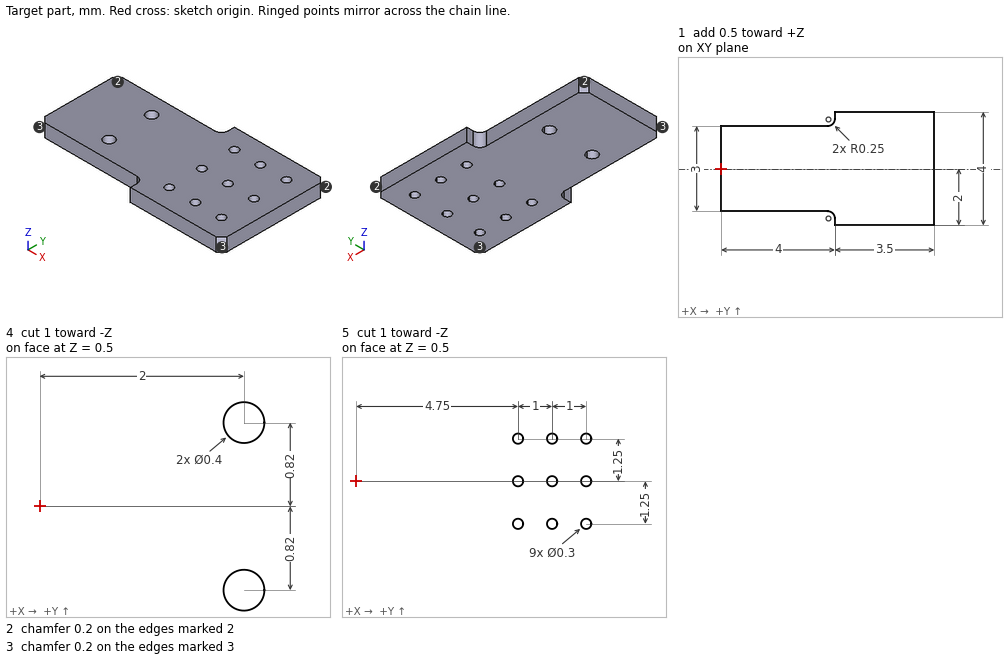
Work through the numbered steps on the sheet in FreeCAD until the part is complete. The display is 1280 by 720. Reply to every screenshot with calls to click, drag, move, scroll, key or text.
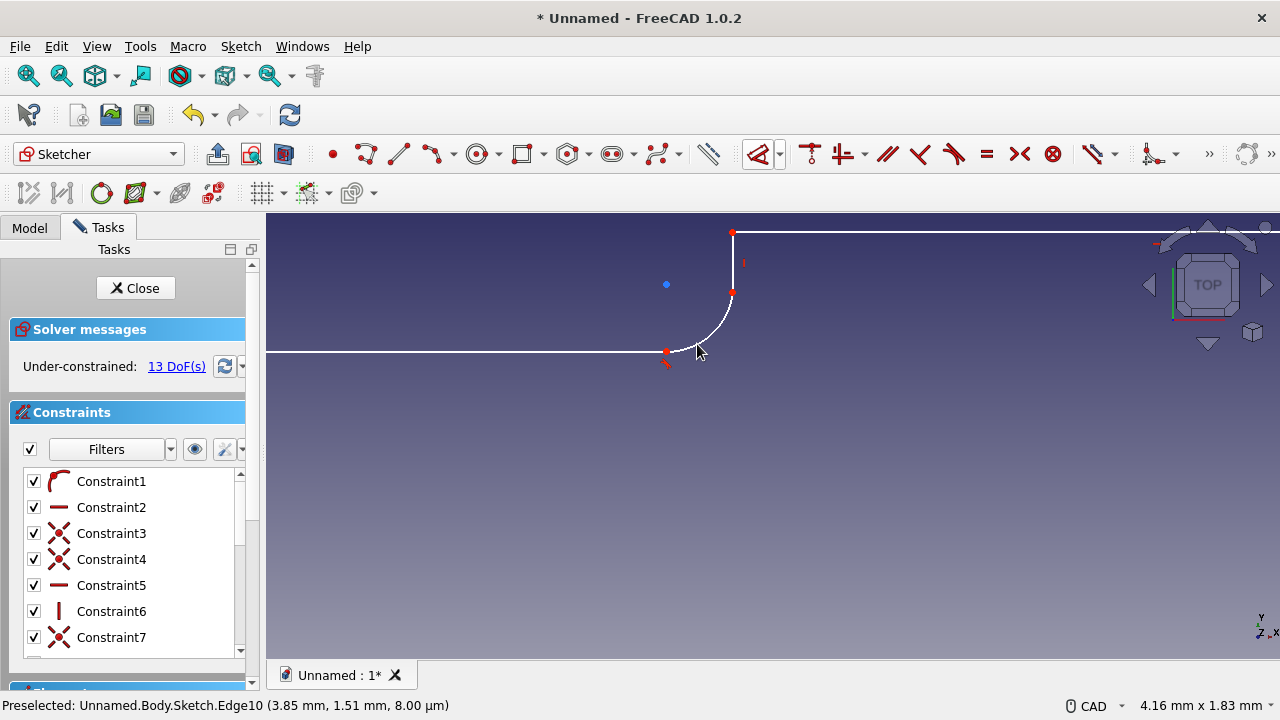
scroll(719, 316, down, 6)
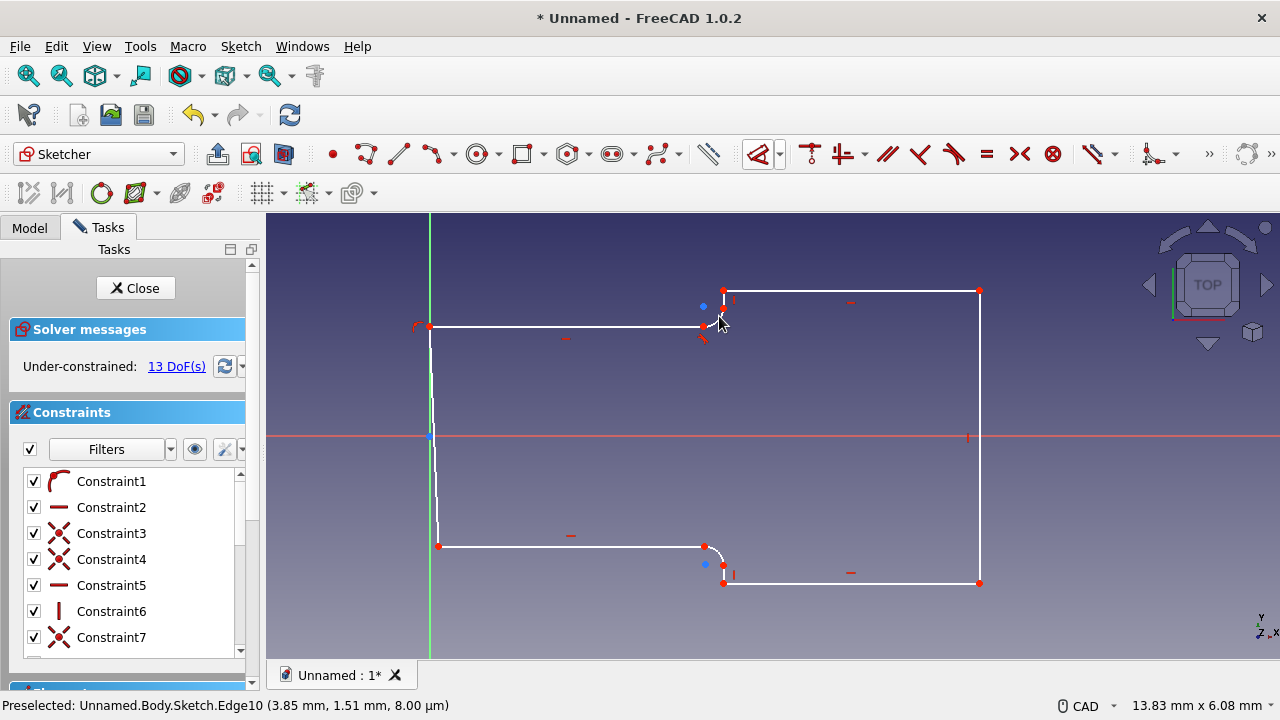
click(518, 547)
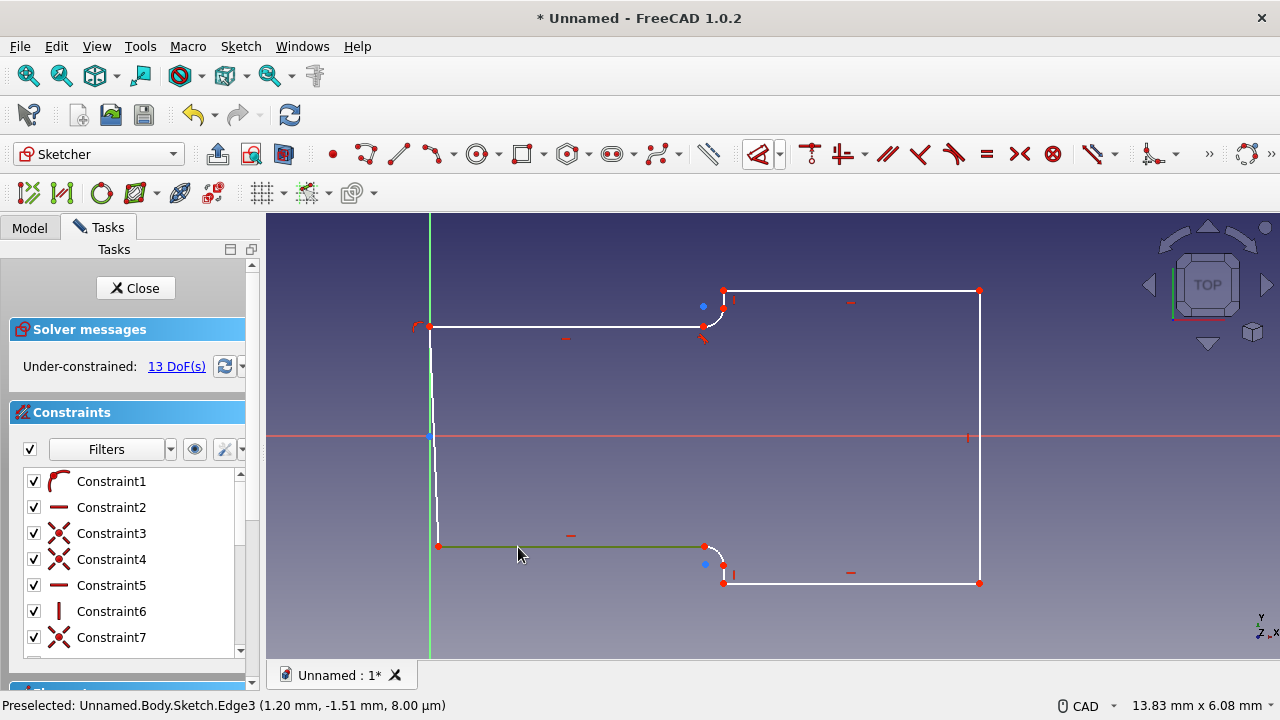
click(718, 552)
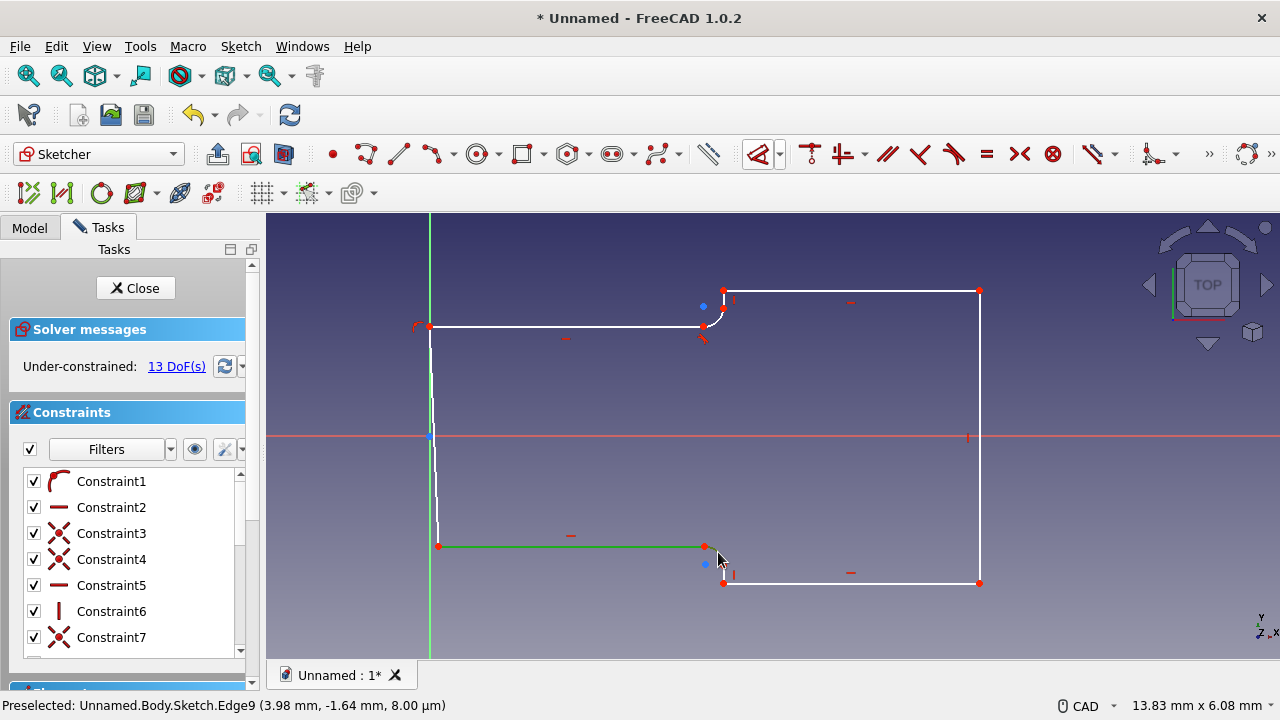
key(t)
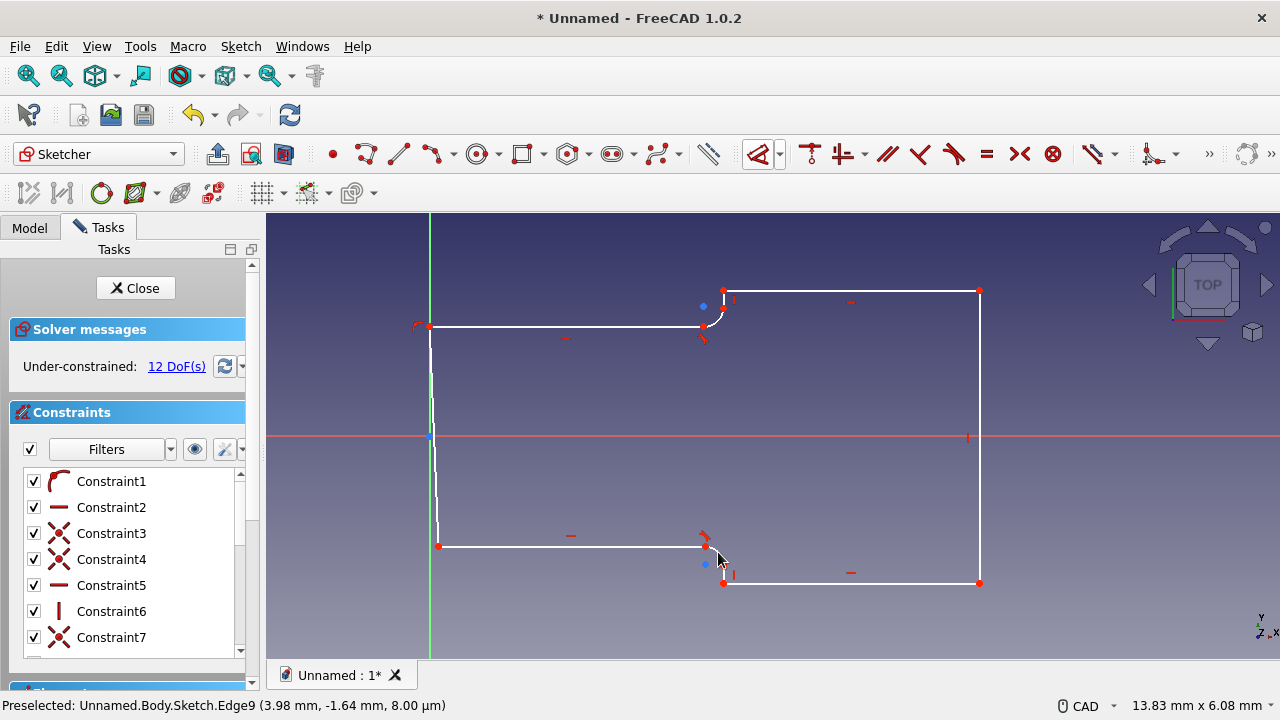
scroll(724, 575, up, 3)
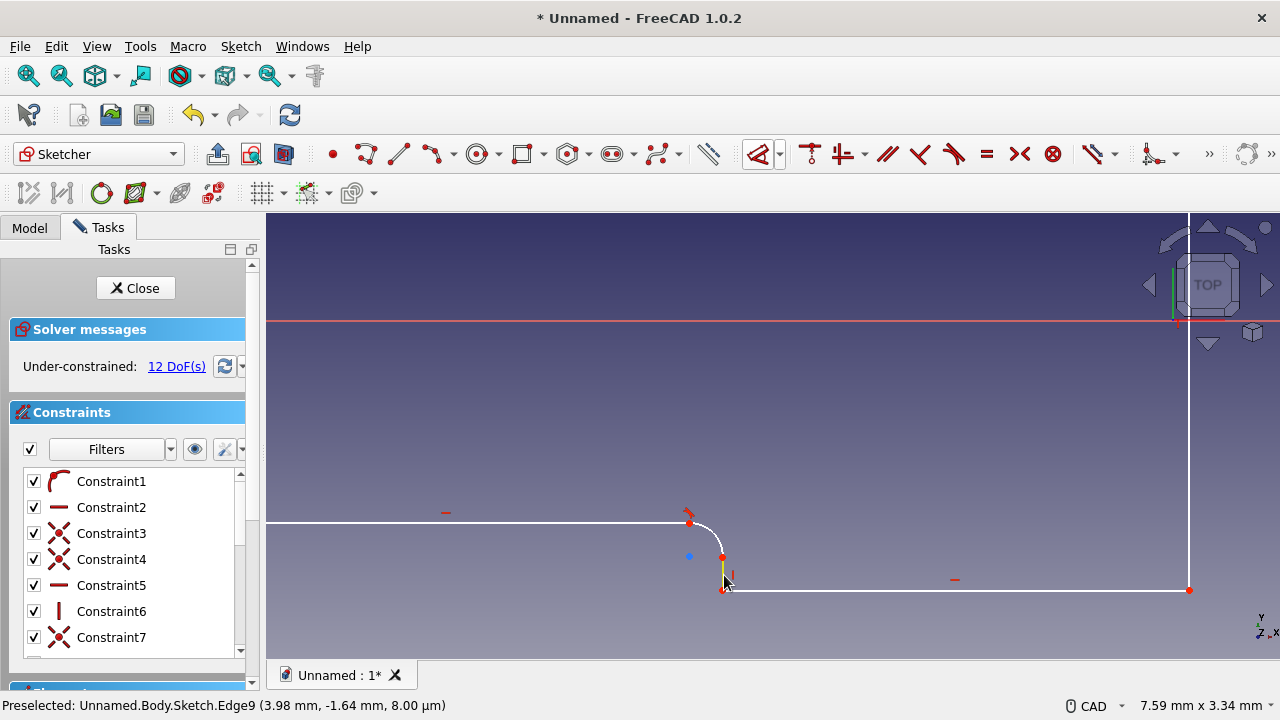
click(723, 574)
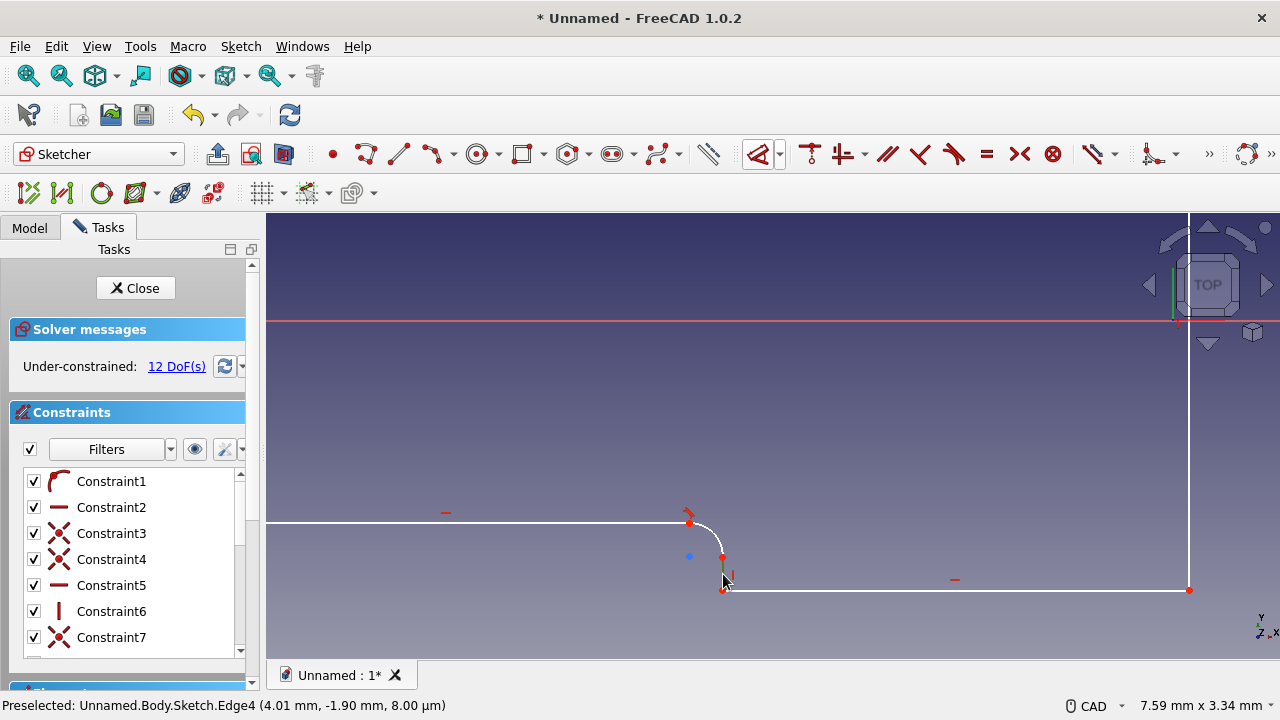
click(720, 542)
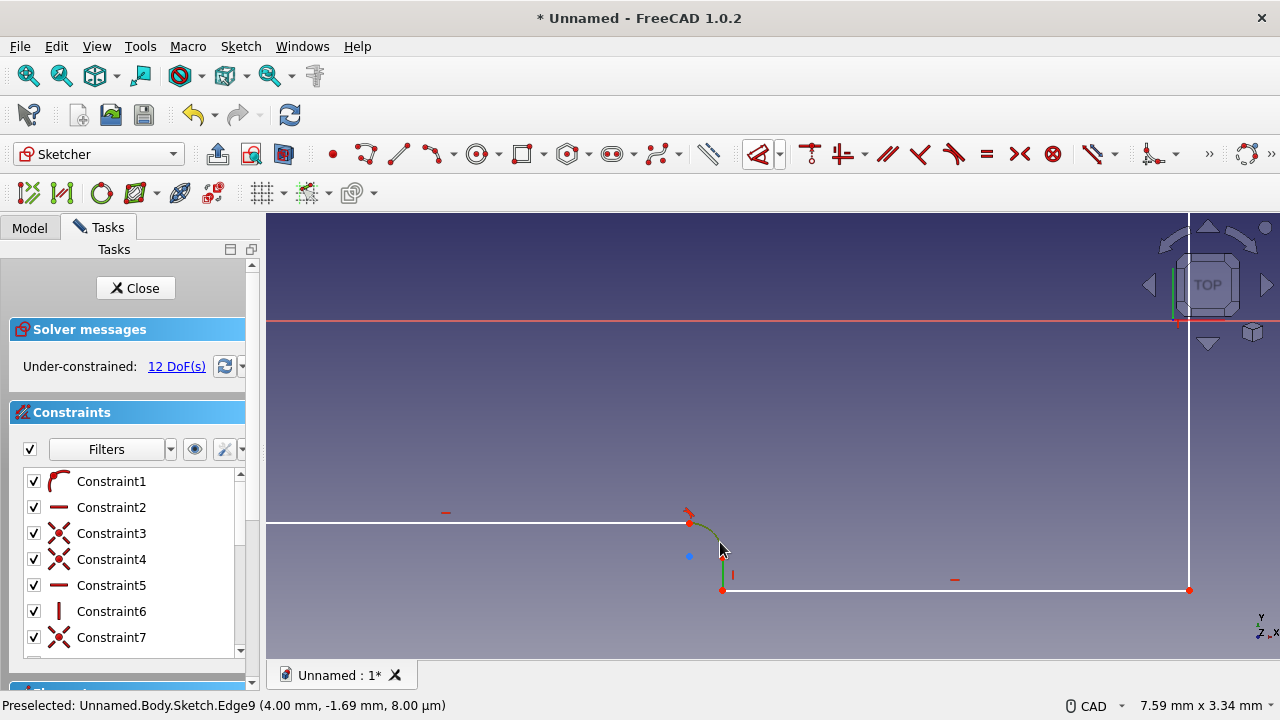
key(t)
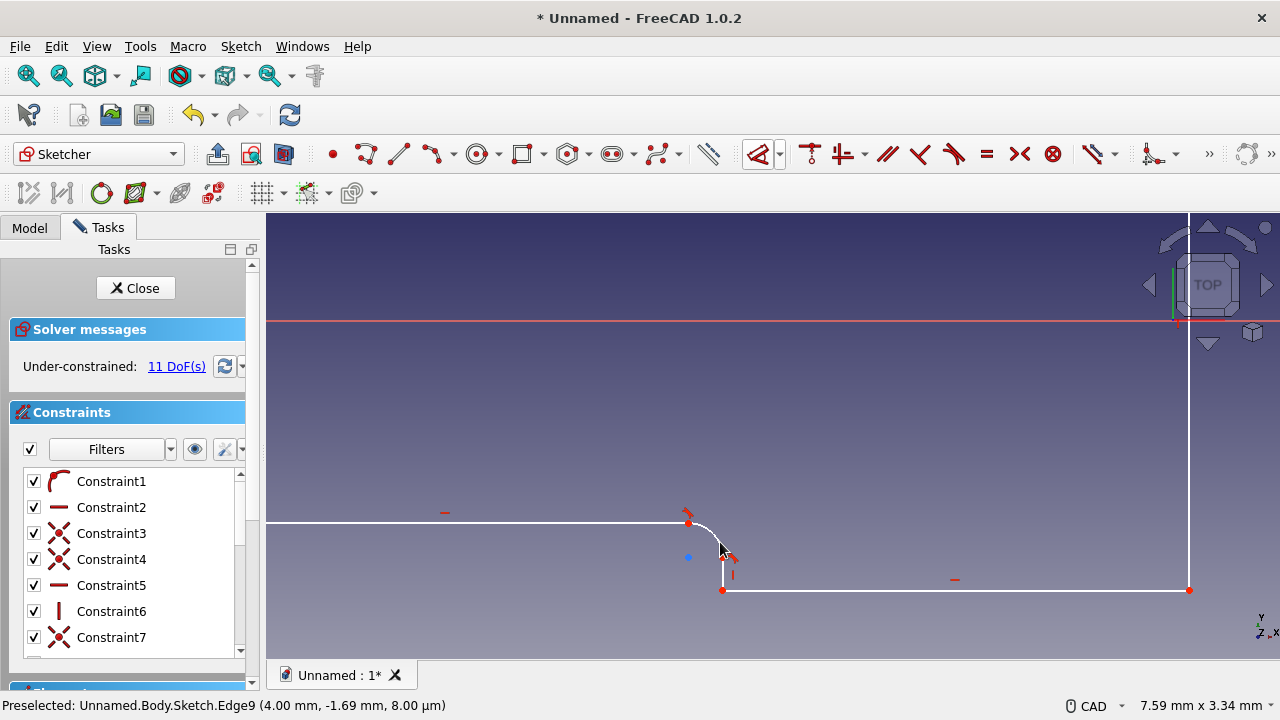
scroll(724, 575, down, 3)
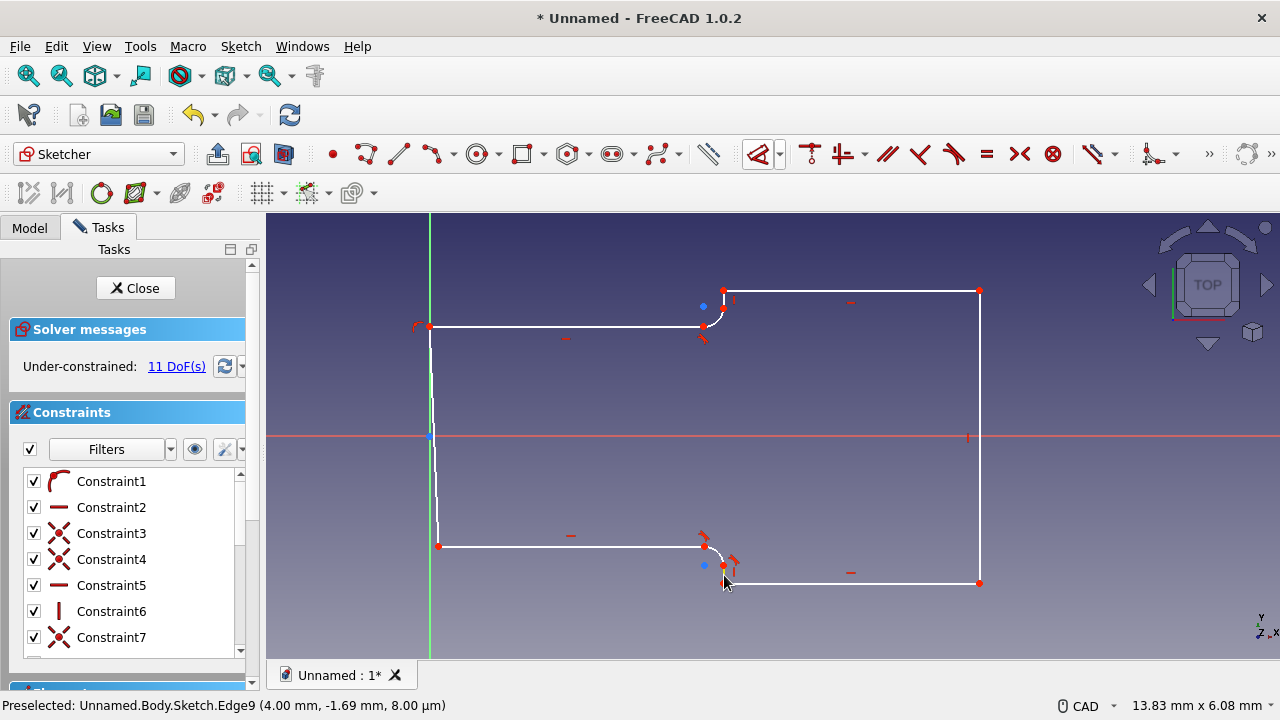
scroll(724, 296, up, 5)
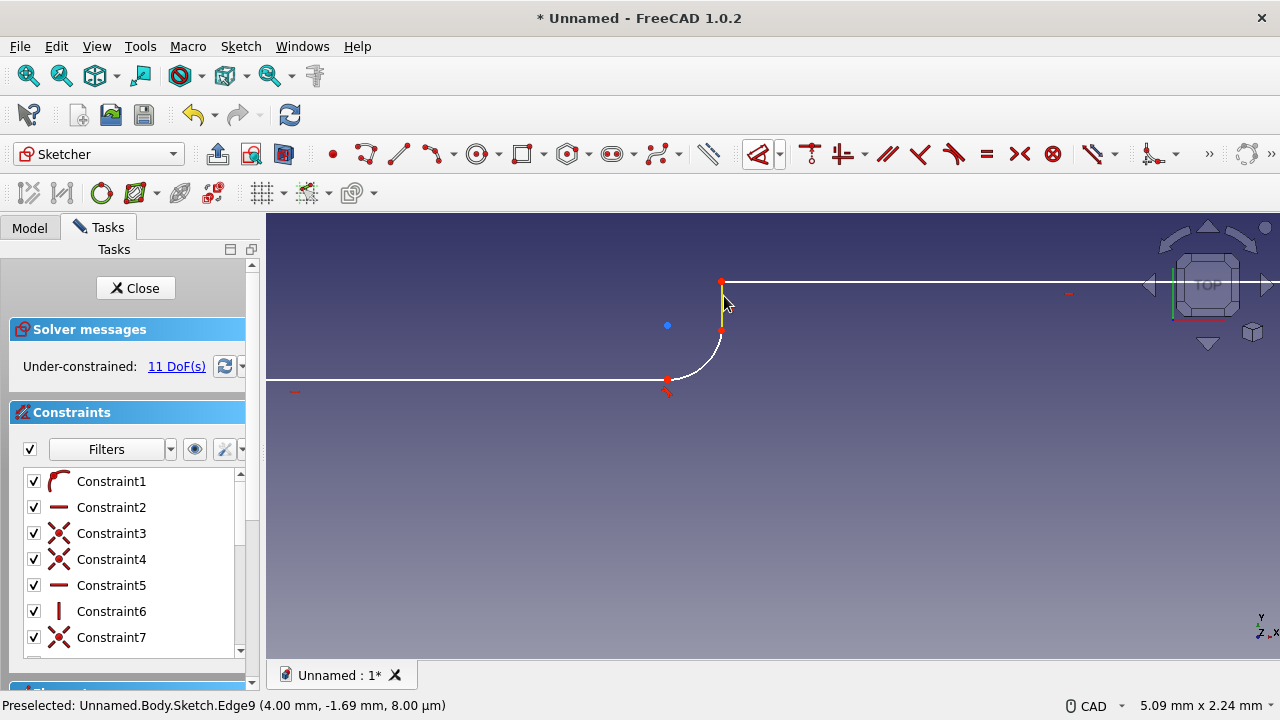
click(722, 297)